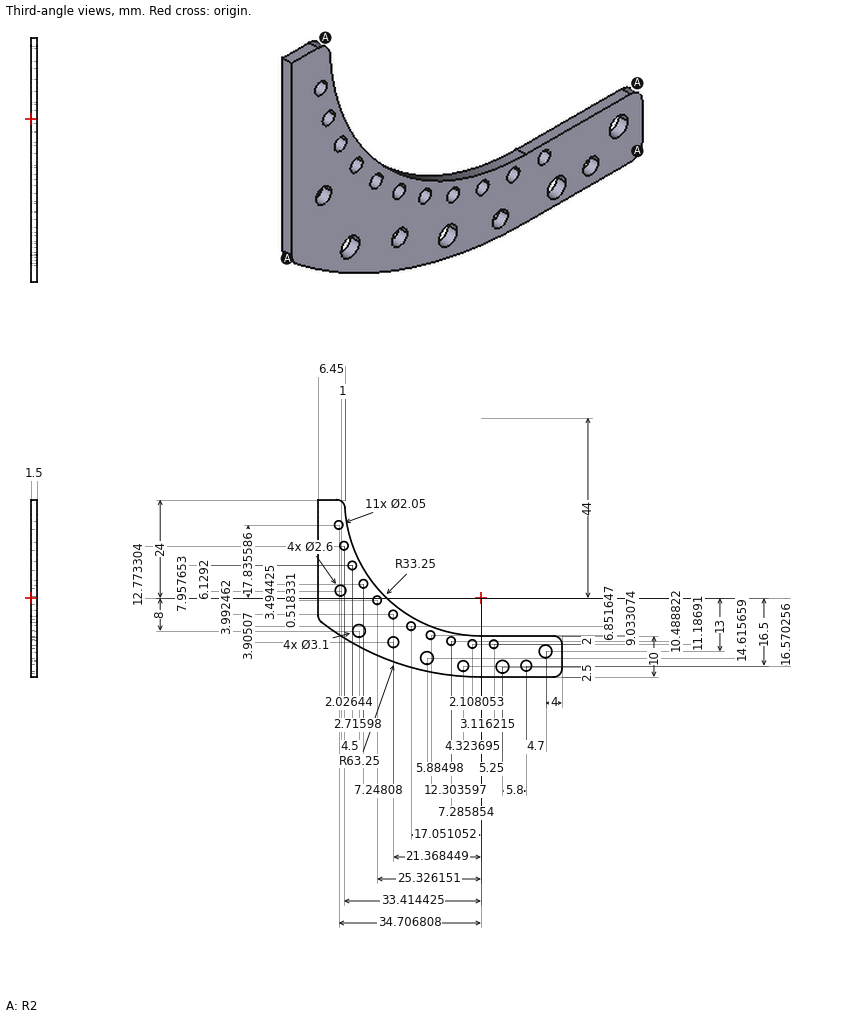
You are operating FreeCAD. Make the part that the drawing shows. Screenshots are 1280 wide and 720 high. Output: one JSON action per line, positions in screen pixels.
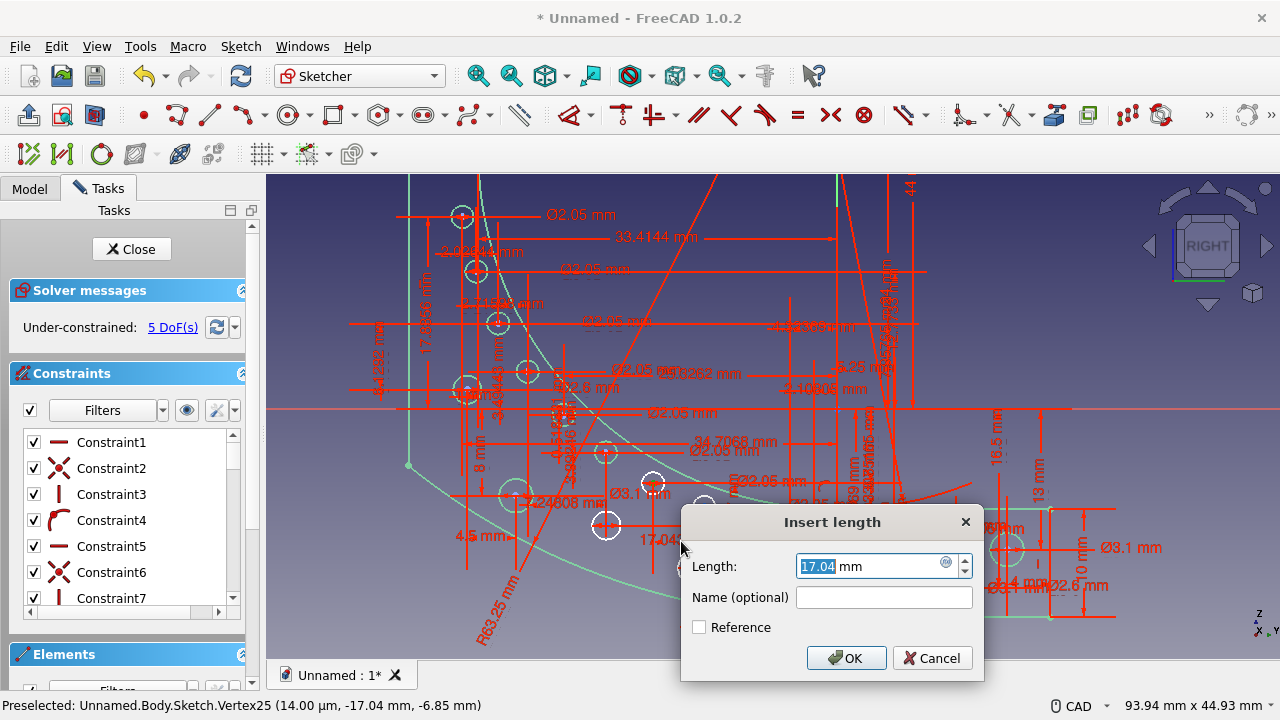
{"action": "type", "text": "17.051052"}
{"action": "key", "text": "Return"}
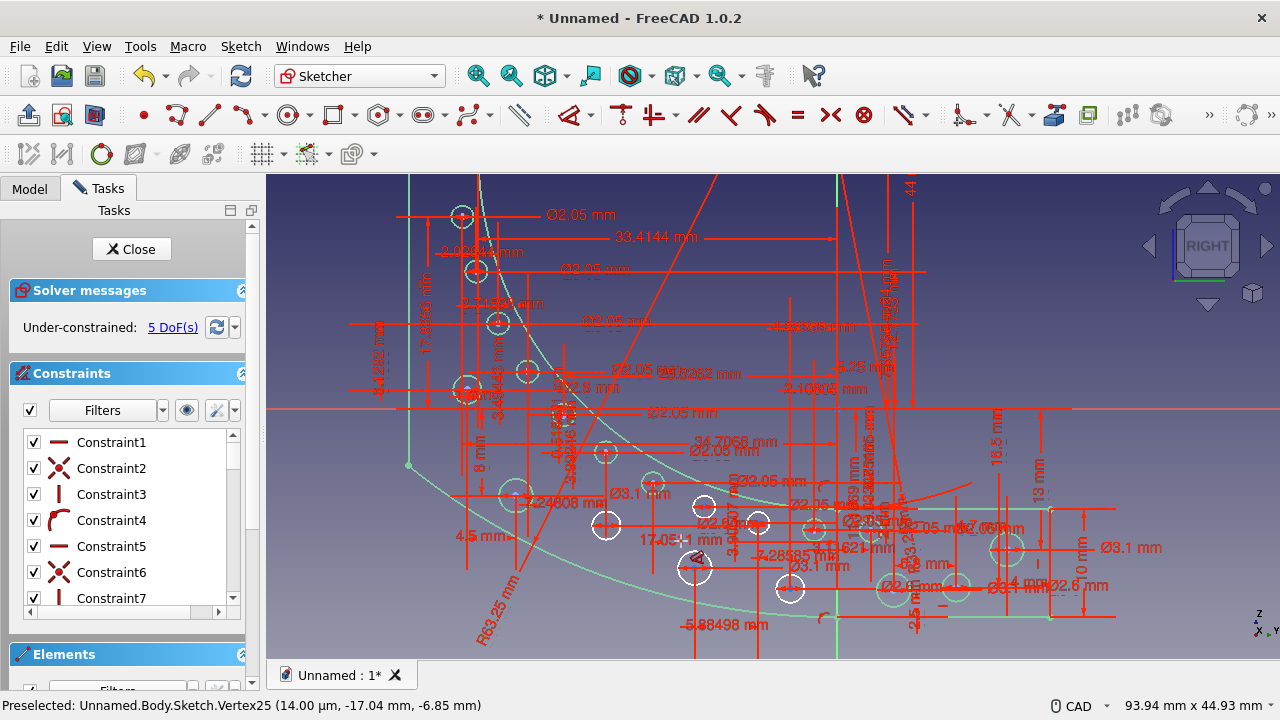
{"action": "left_click", "coordinate": [606, 526]}
{"action": "left_click", "coordinate": [722, 584]}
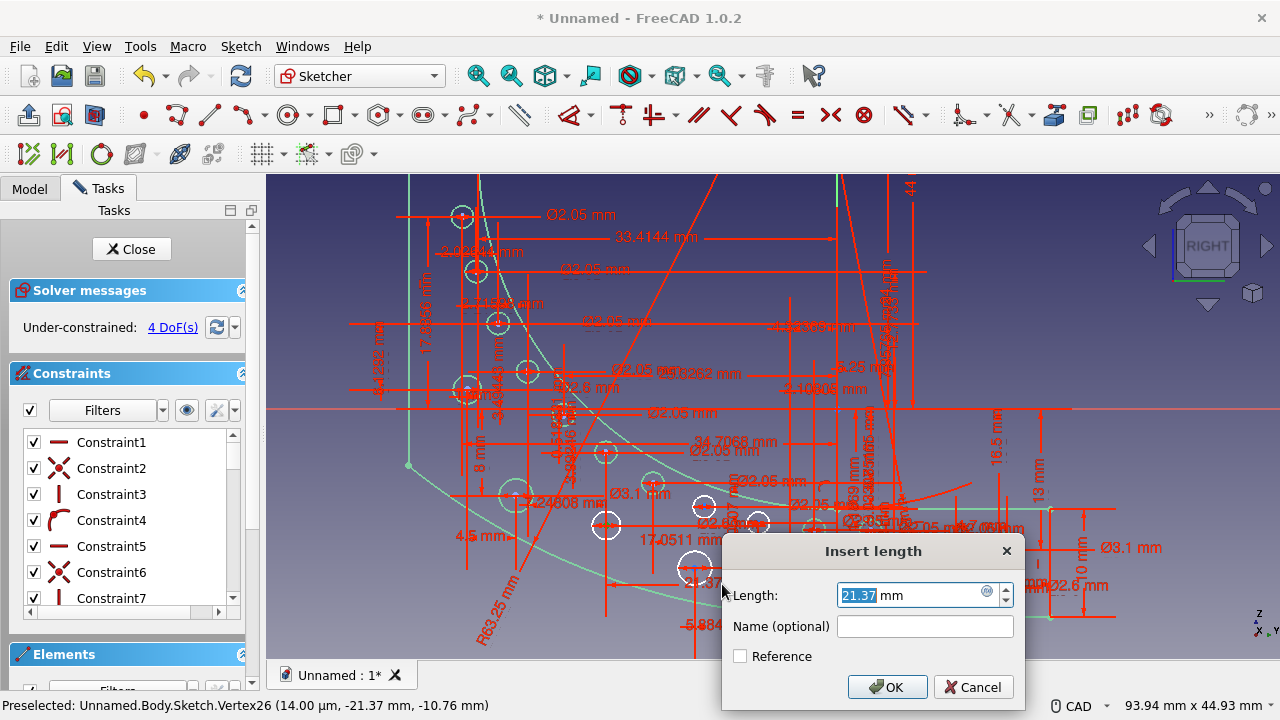
{"action": "type", "text": "21.368449"}
{"action": "key", "text": "Return"}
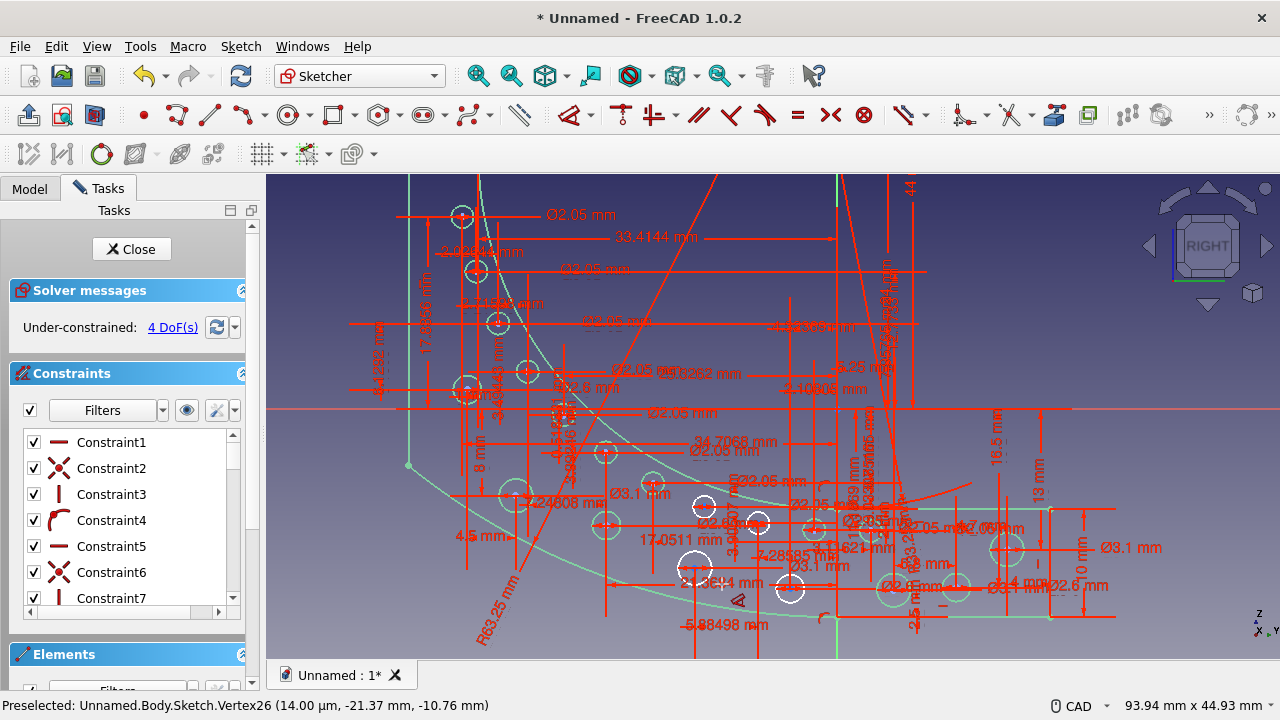
{"action": "left_click", "coordinate": [704, 507]}
{"action": "left_click", "coordinate": [771, 351]}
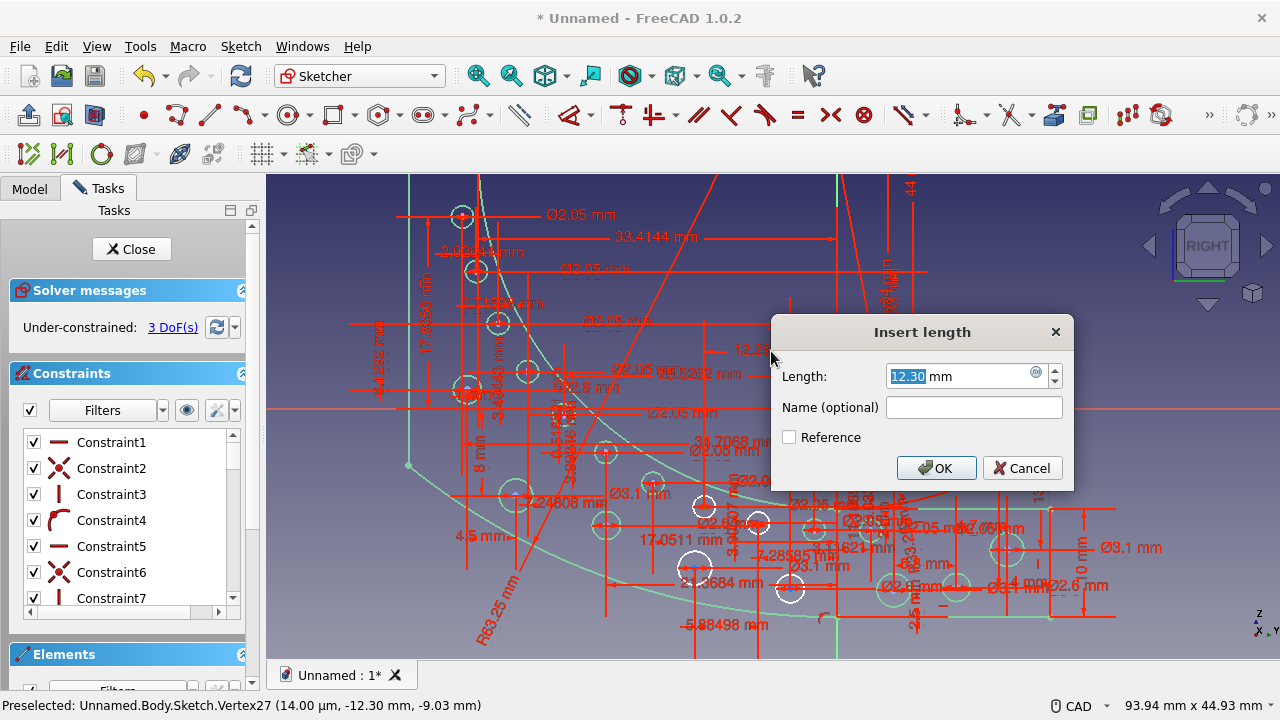
{"action": "type", "text": "12.303597"}
{"action": "key", "text": "Return"}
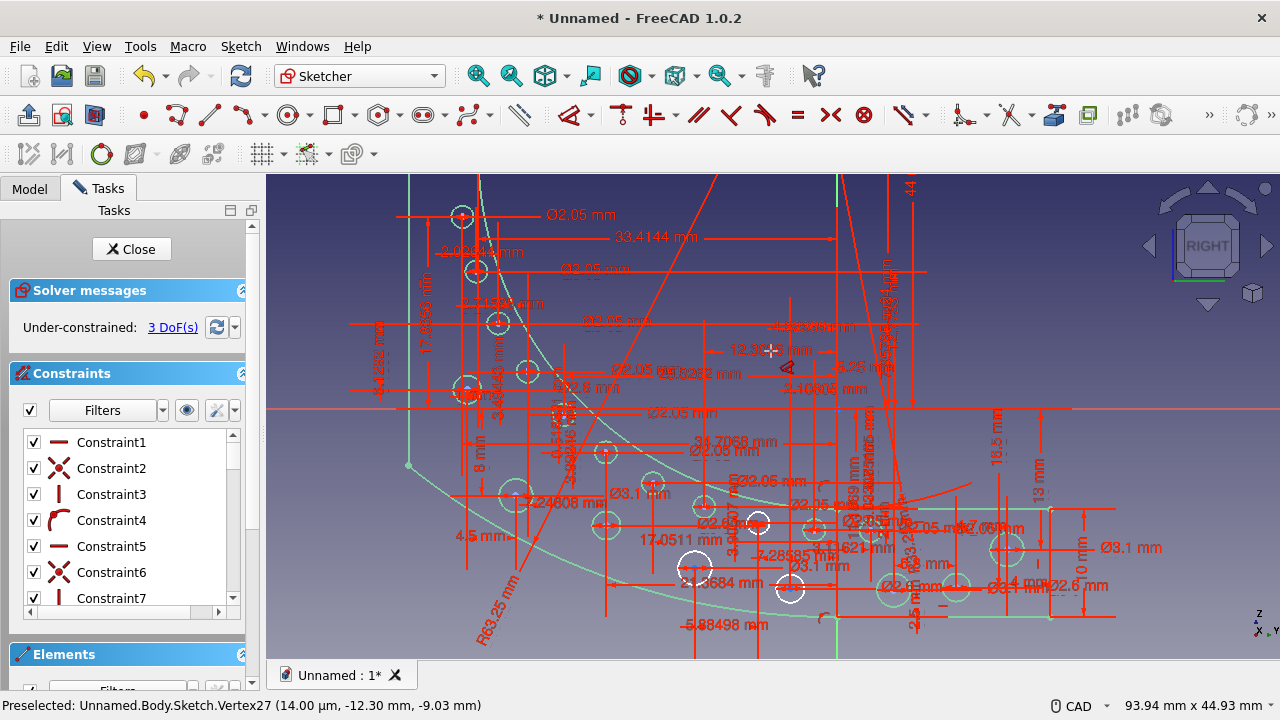
{"action": "left_click", "coordinate": [695, 568]}
{"action": "left_click", "coordinate": [661, 433]}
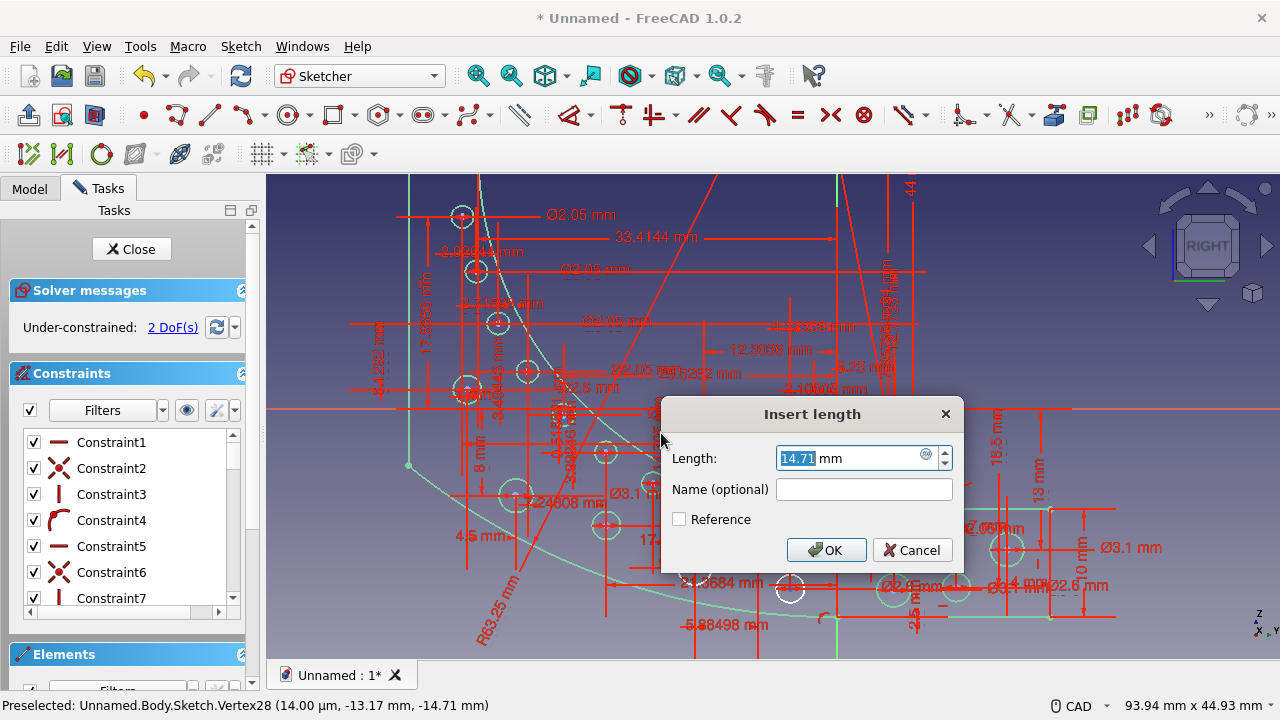
{"action": "type", "text": "14.615659"}
{"action": "key", "text": "Return"}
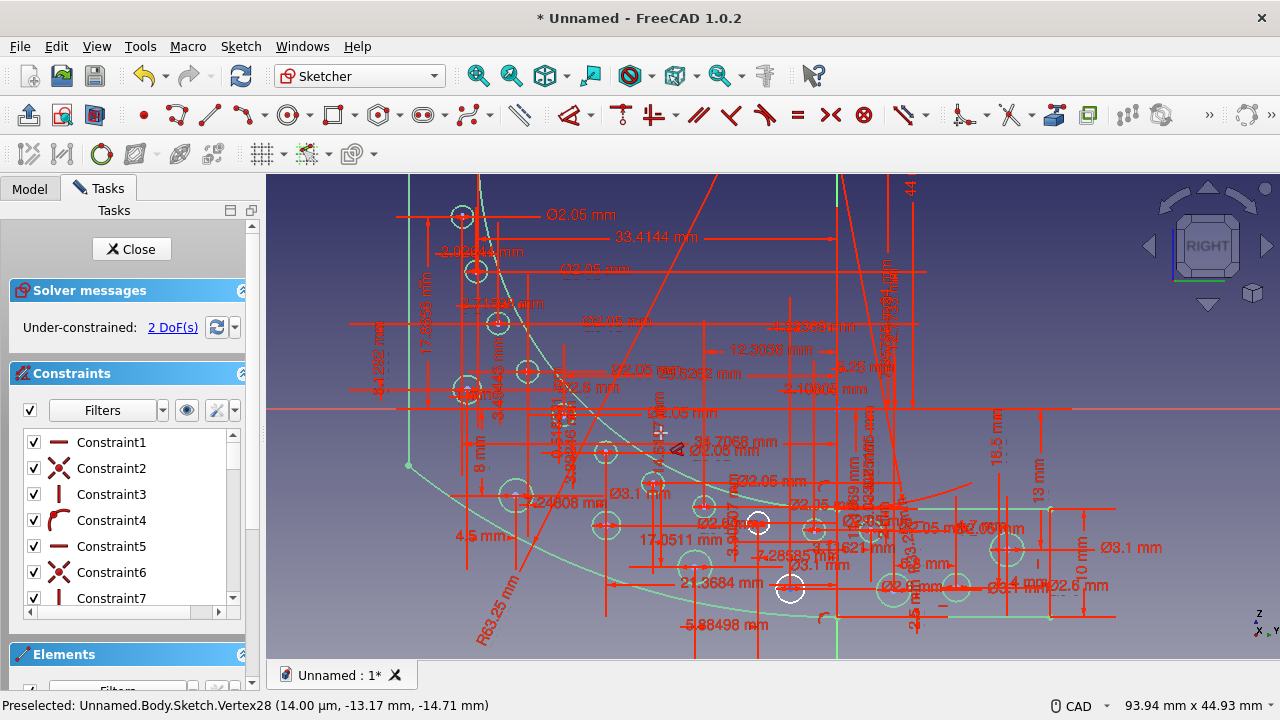
{"action": "left_click", "coordinate": [758, 523]}
{"action": "left_click", "coordinate": [871, 426]}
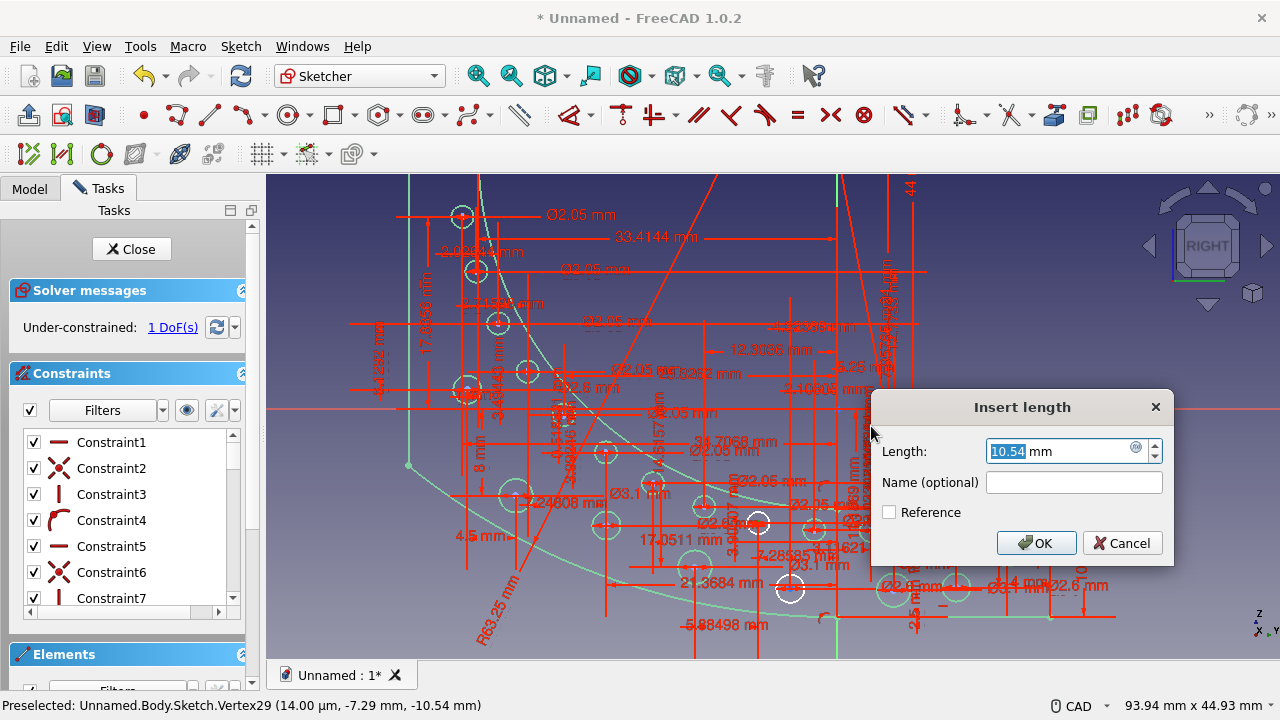
{"action": "type", "text": "10.488822"}
{"action": "key", "text": "Return"}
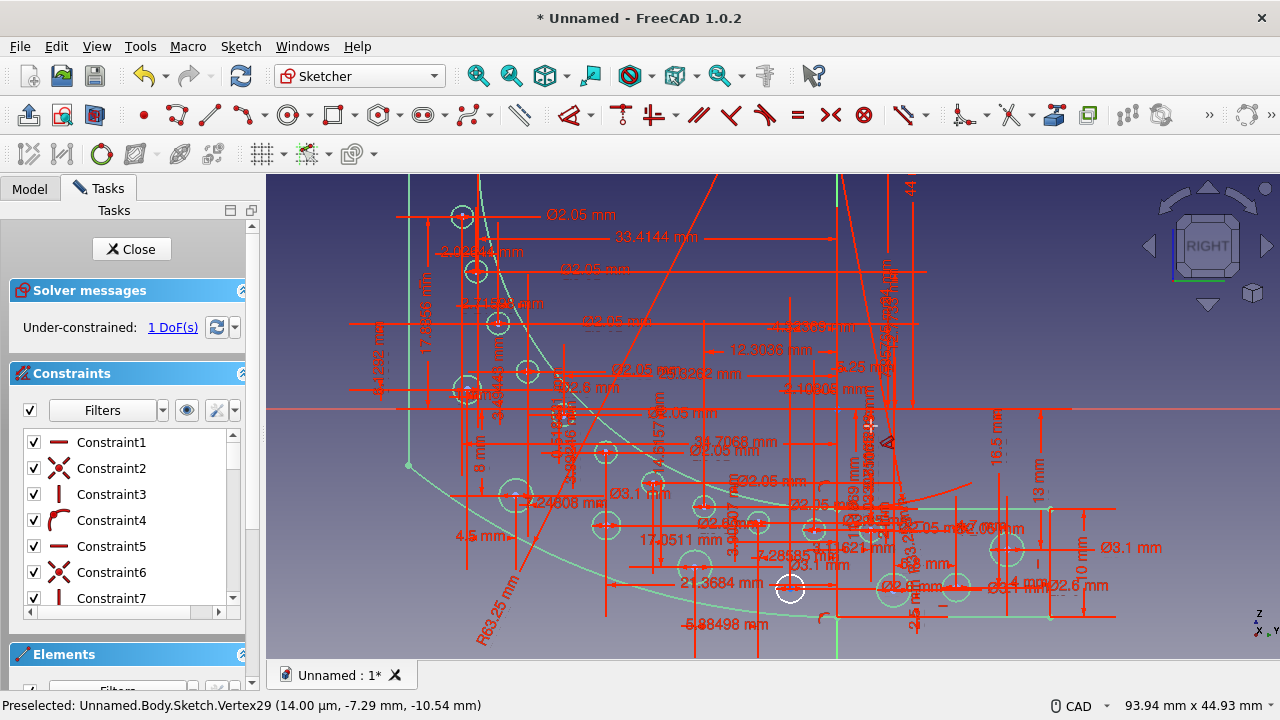
{"action": "left_click", "coordinate": [790, 589]}
{"action": "left_click", "coordinate": [943, 458]}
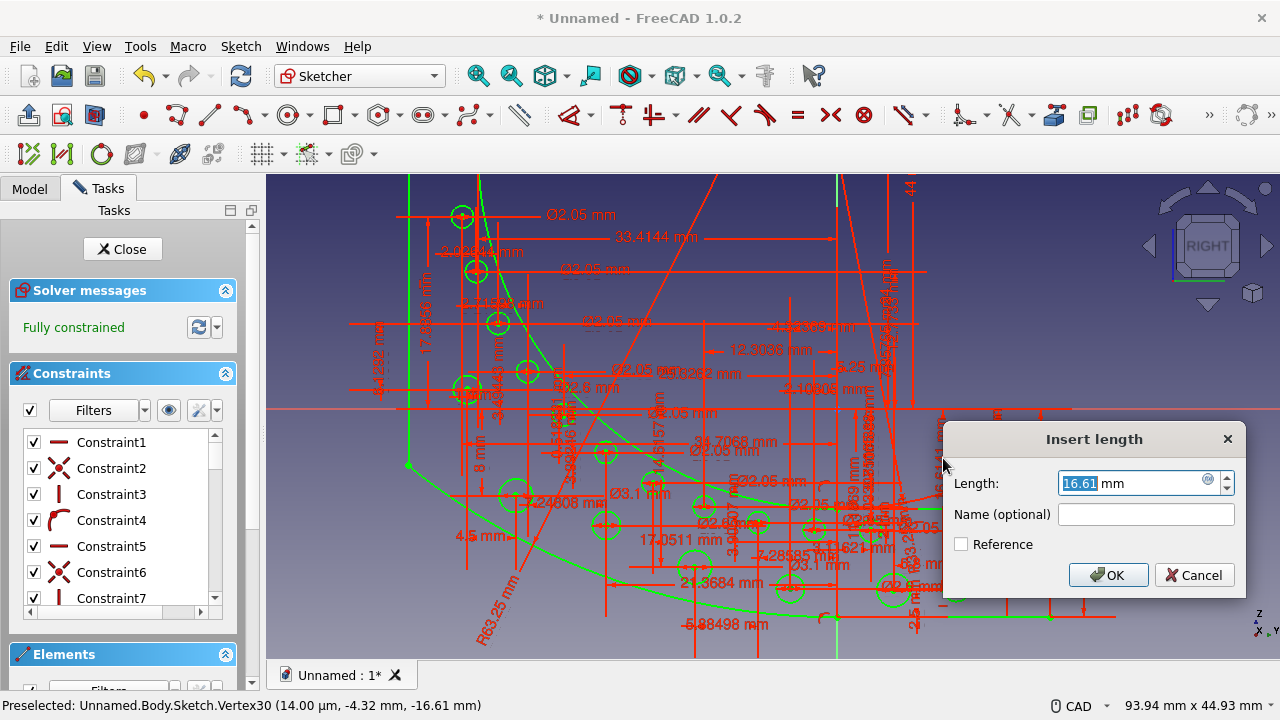
{"action": "type", "text": "16.570256"}
{"action": "key", "text": "Return"}
{"action": "key", "text": "Escape"}